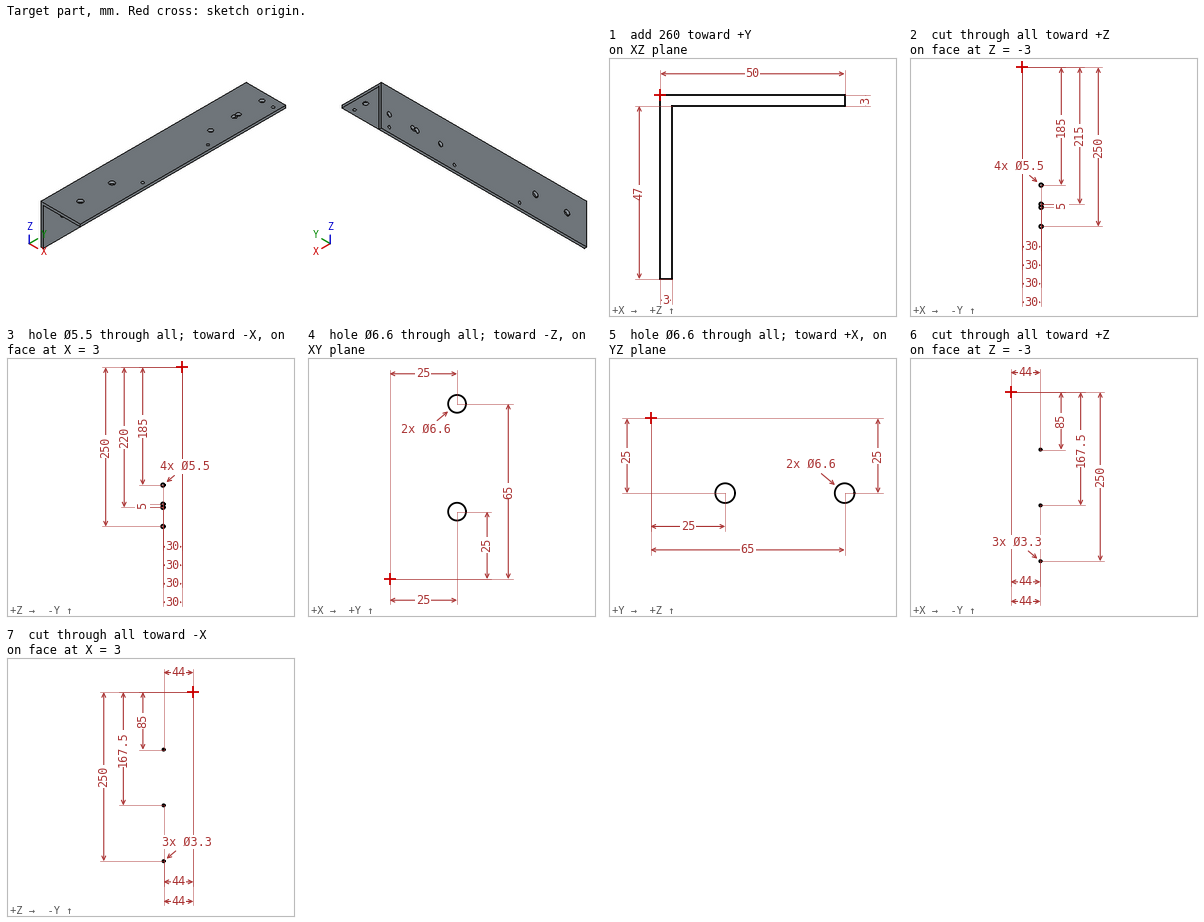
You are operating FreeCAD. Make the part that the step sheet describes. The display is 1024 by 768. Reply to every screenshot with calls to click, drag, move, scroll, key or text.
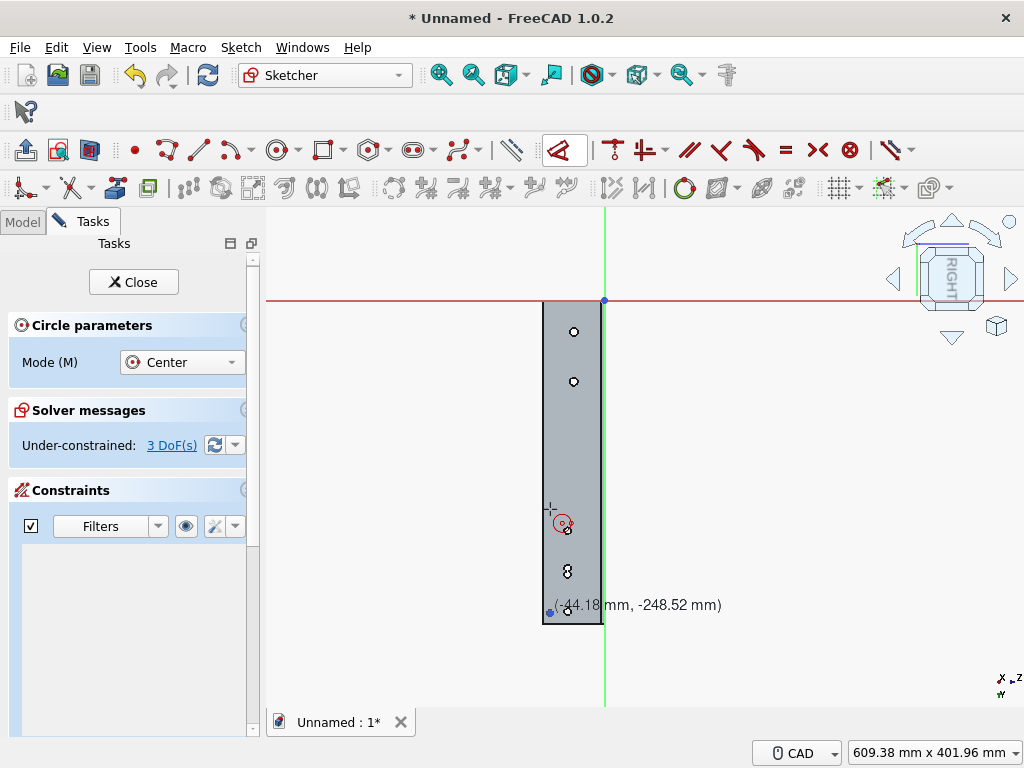
click(550, 509)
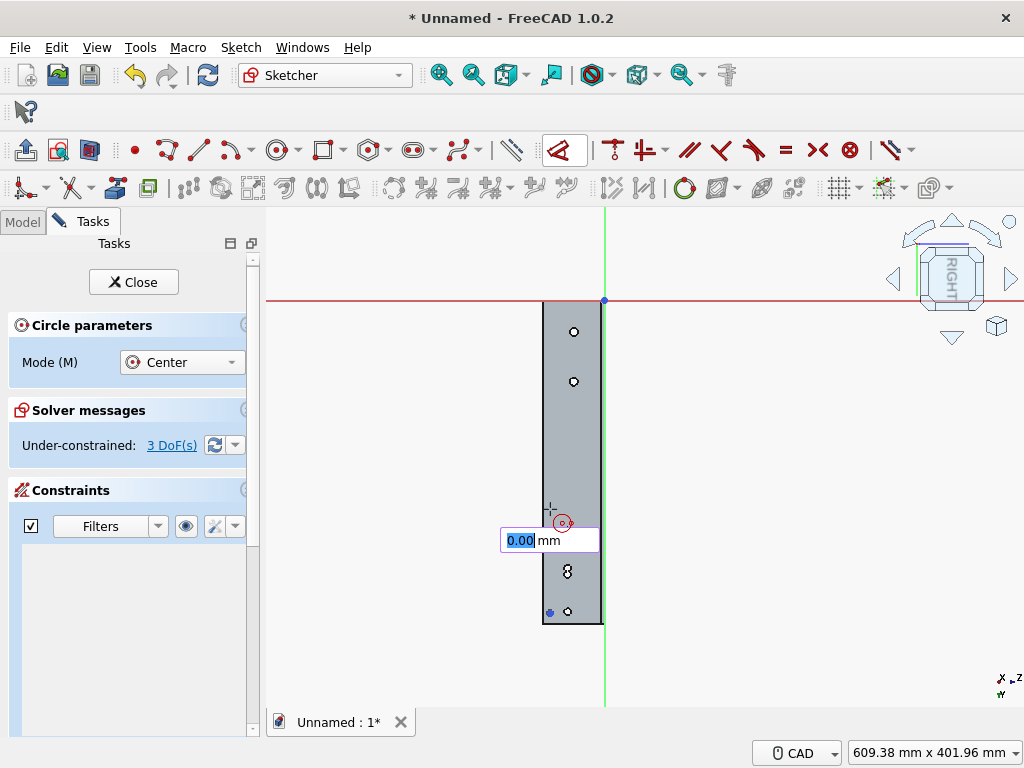
scroll(552, 508, up, 11)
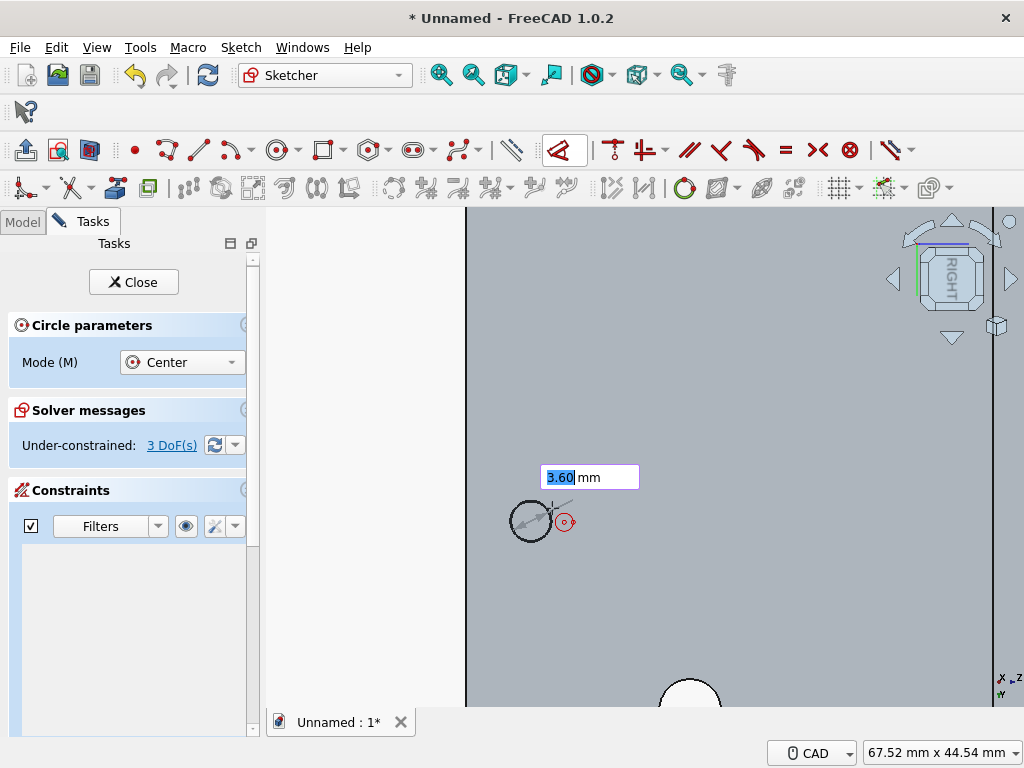
click(546, 500)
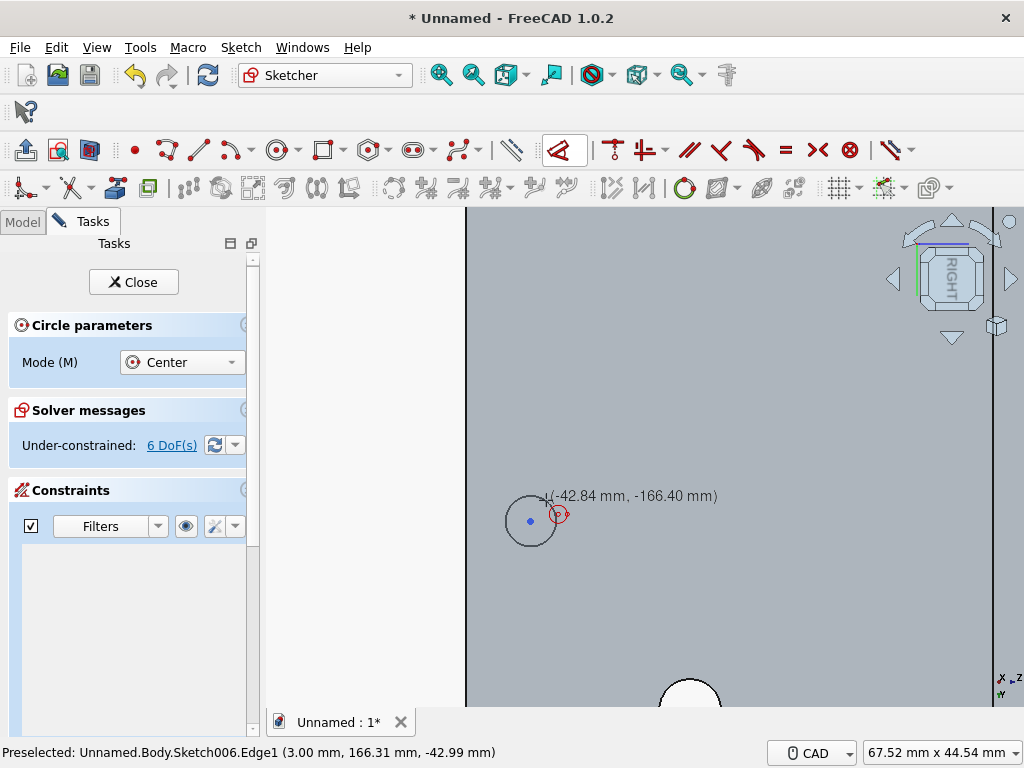
scroll(552, 508, down, 11)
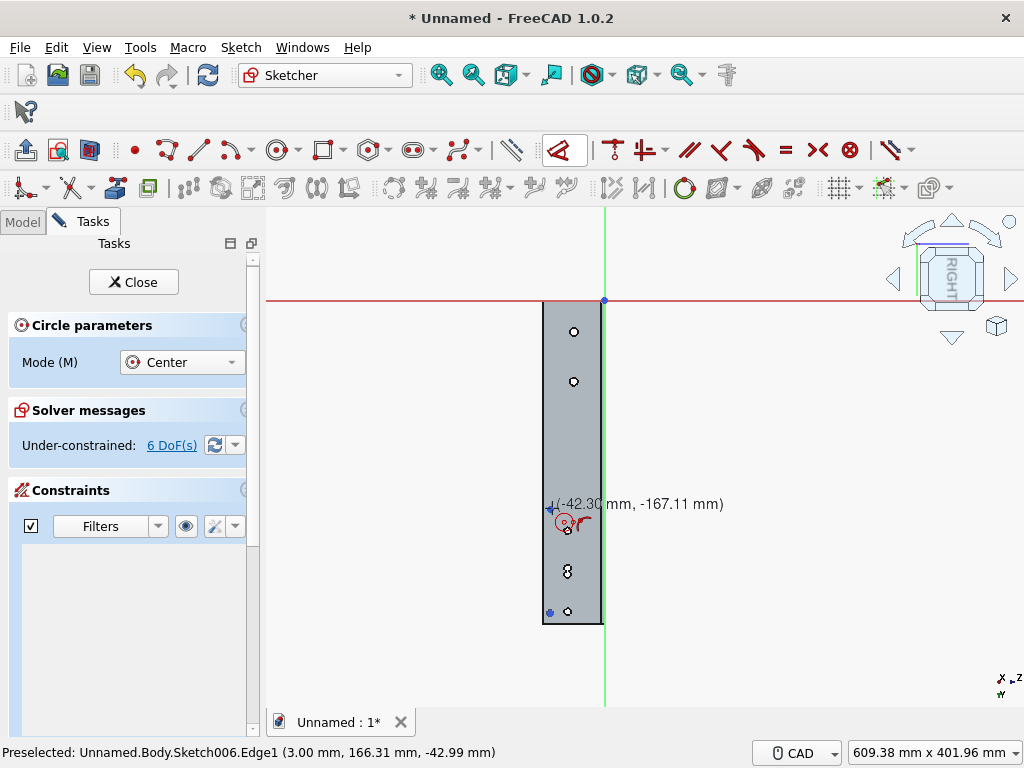
scroll(550, 407, up, 13)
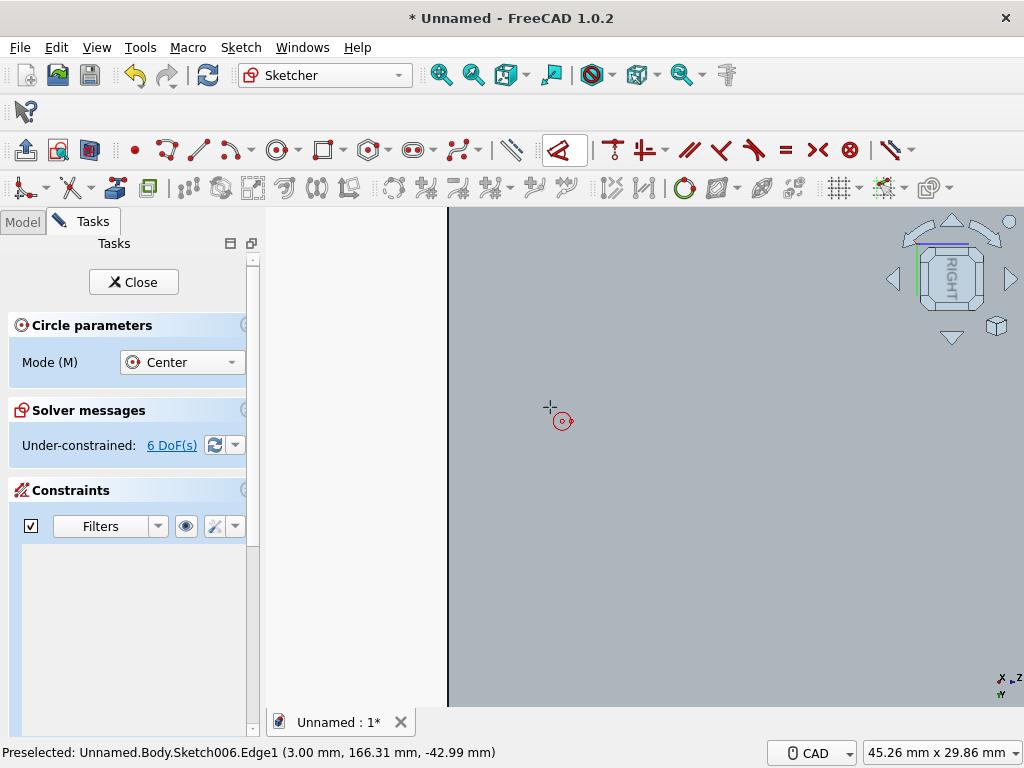
scroll(550, 407, down, 13)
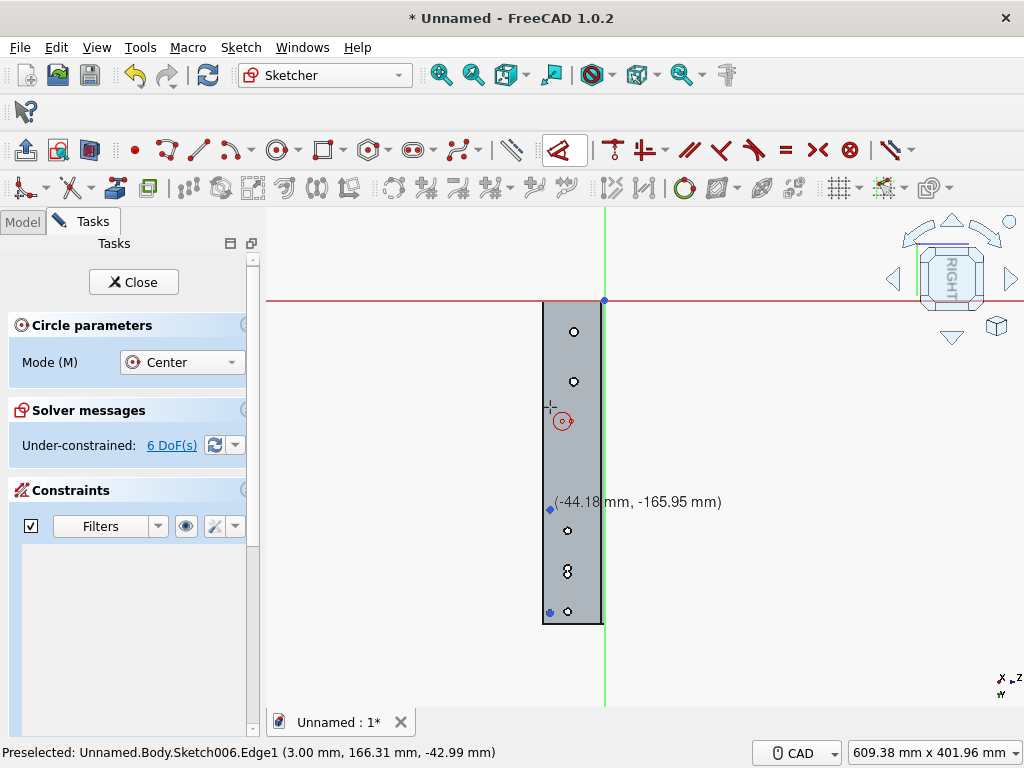
click(550, 407)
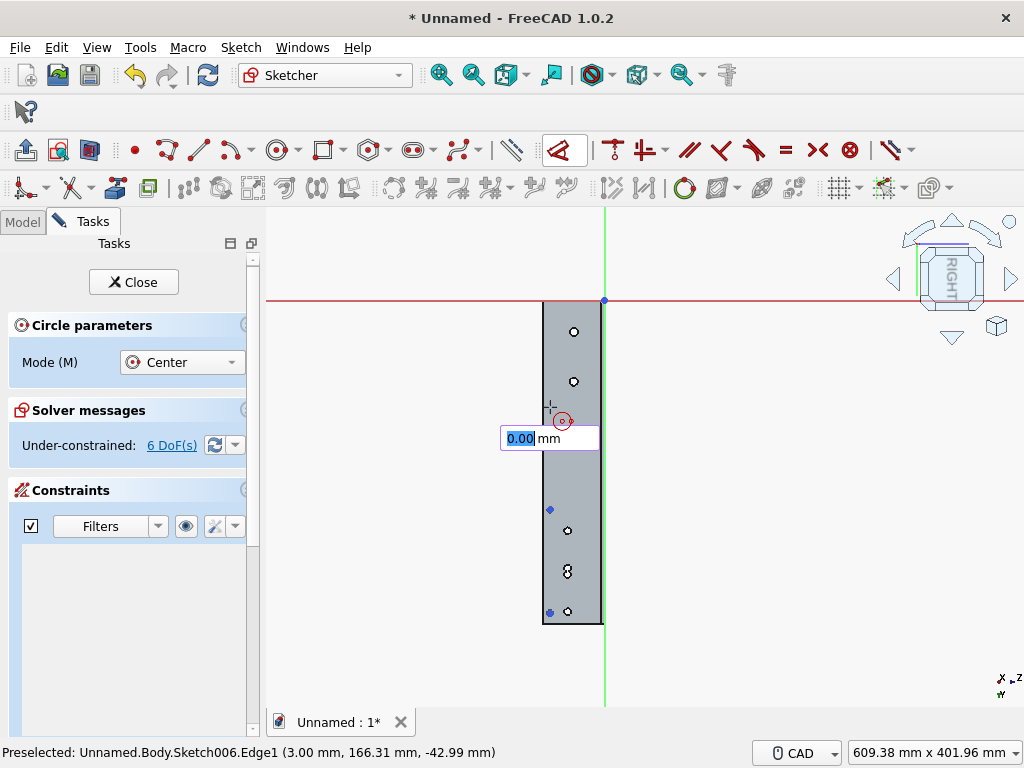
scroll(552, 405, up, 11)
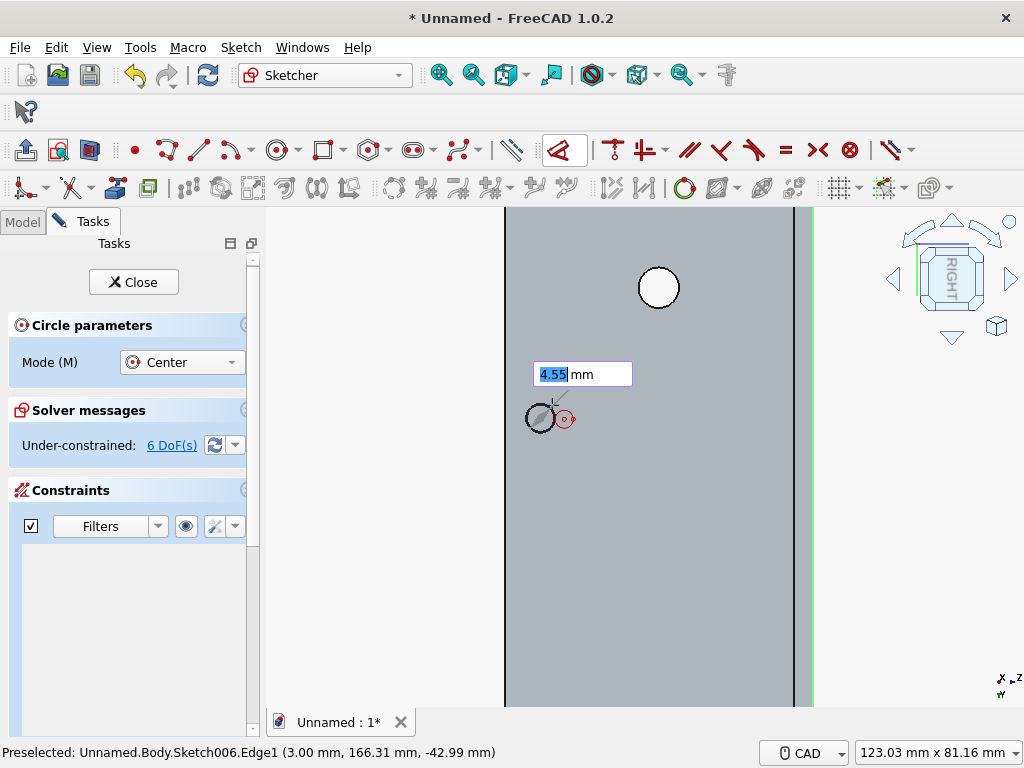
click(546, 402)
key(Escape)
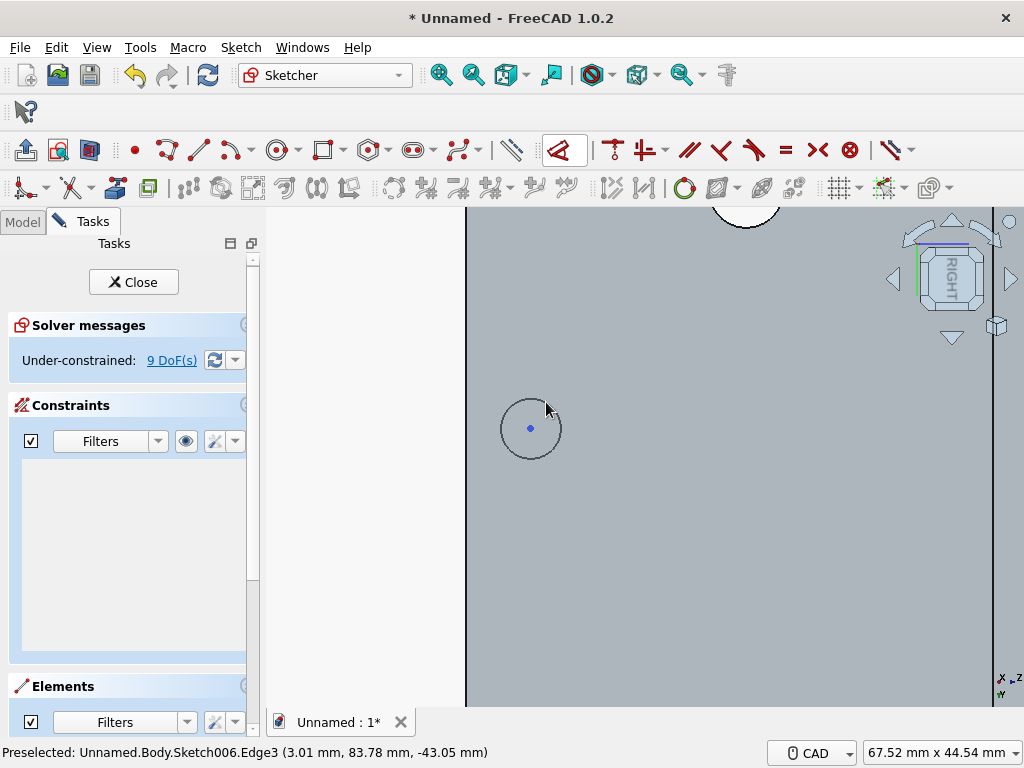
scroll(552, 405, down, 11)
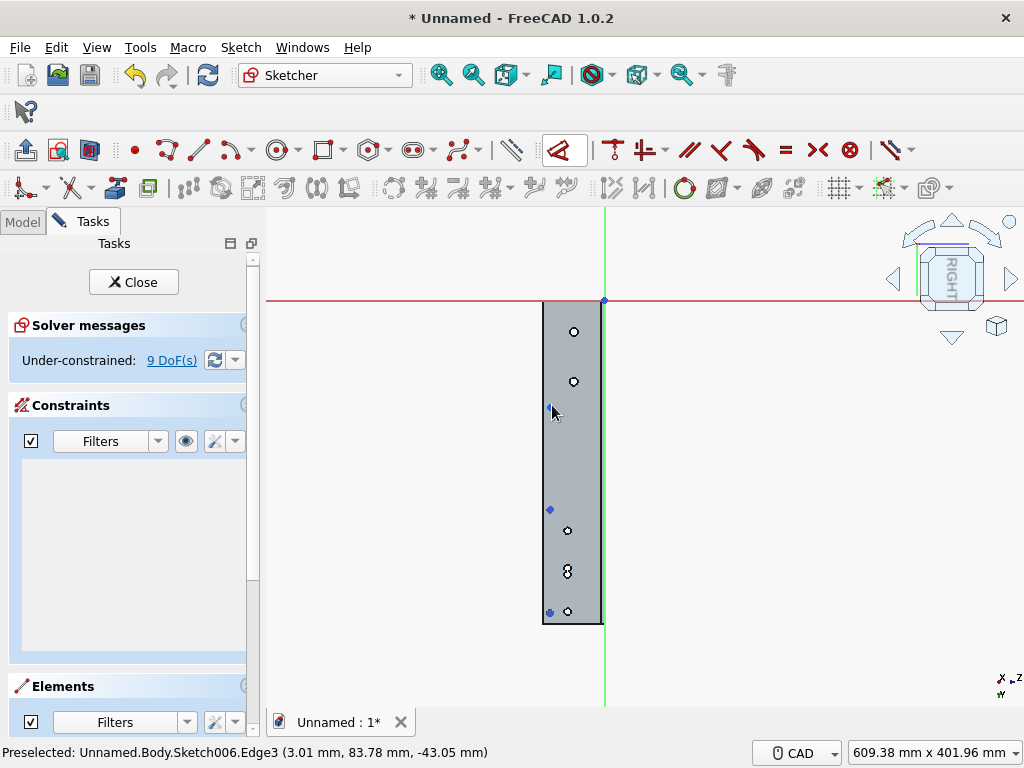
scroll(552, 611, up, 8)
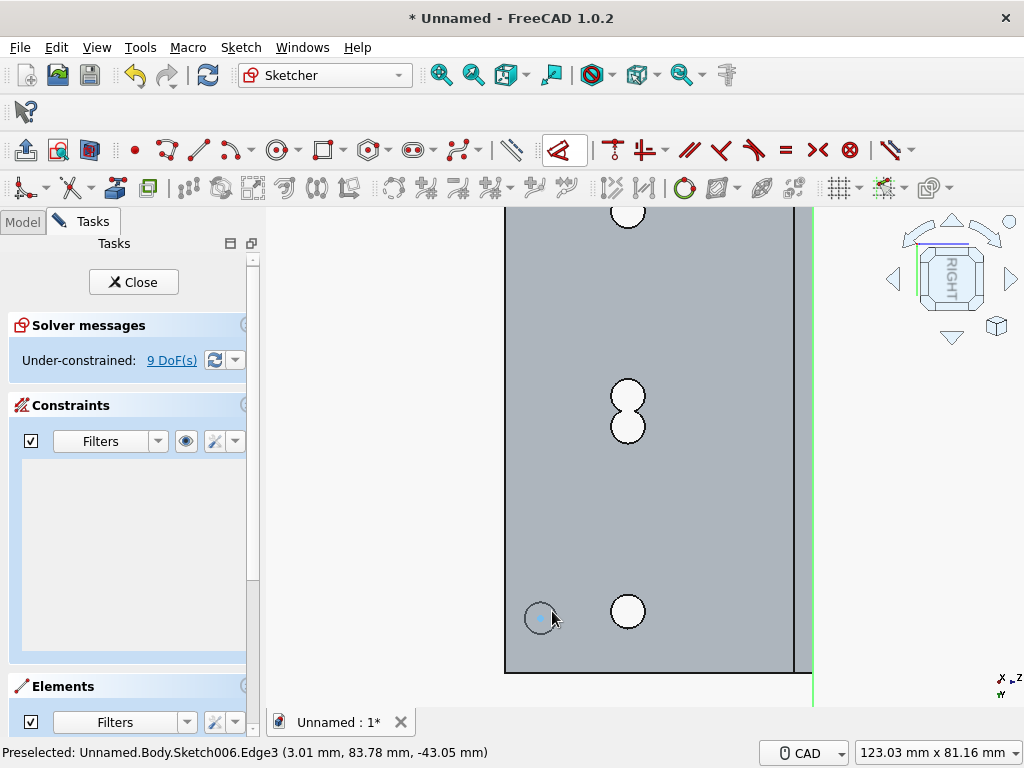
click(552, 607)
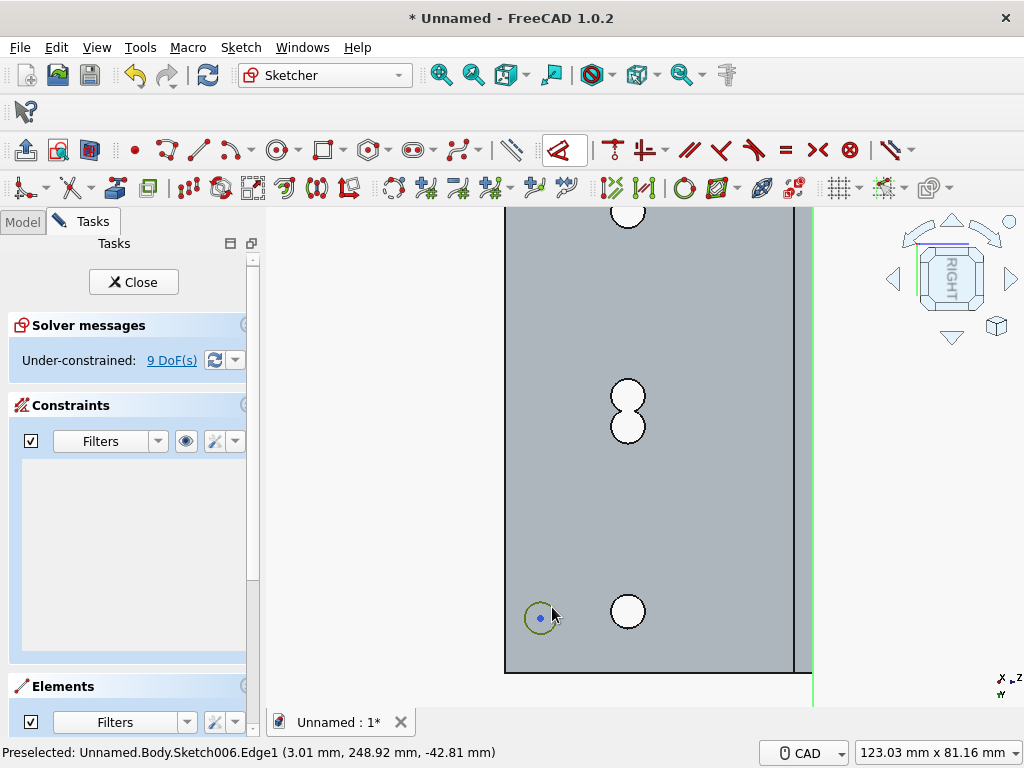
scroll(552, 611, down, 8)